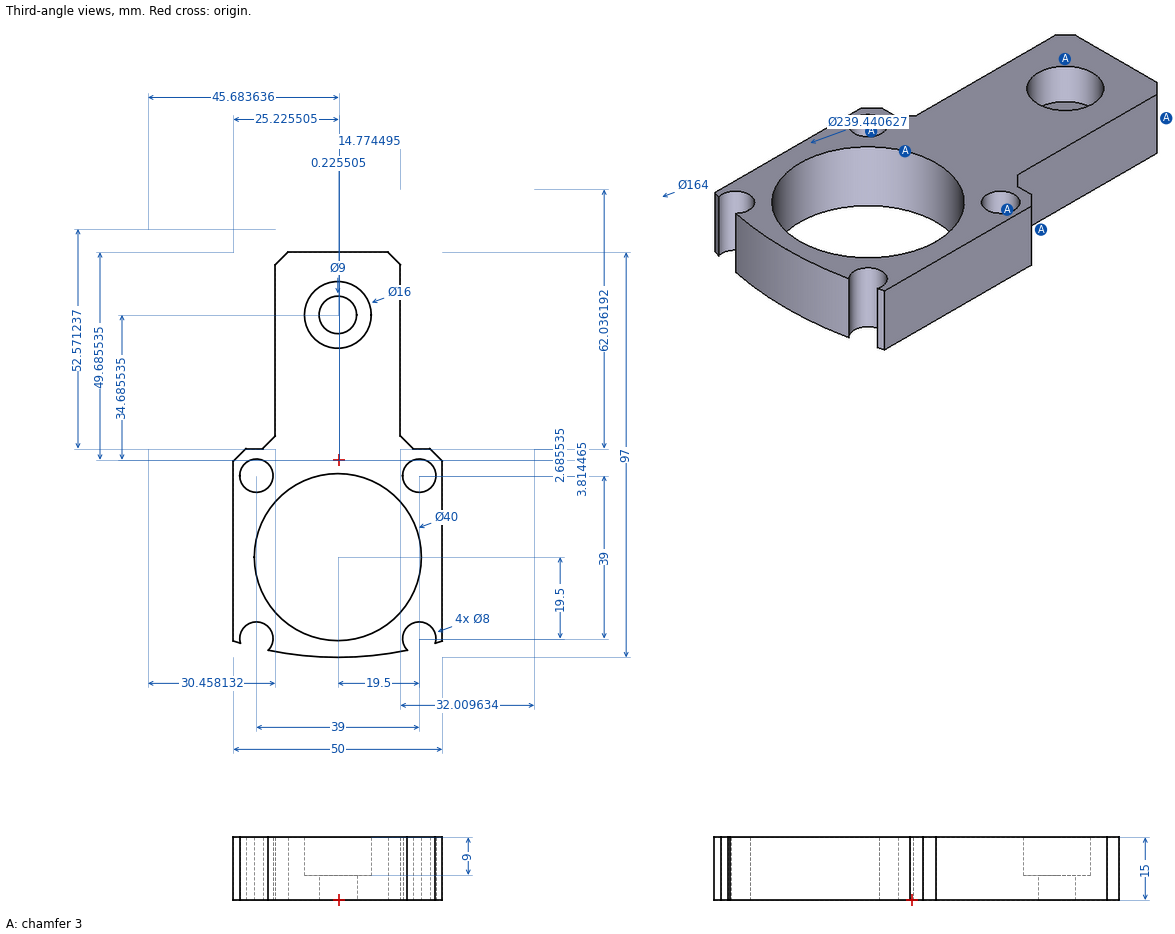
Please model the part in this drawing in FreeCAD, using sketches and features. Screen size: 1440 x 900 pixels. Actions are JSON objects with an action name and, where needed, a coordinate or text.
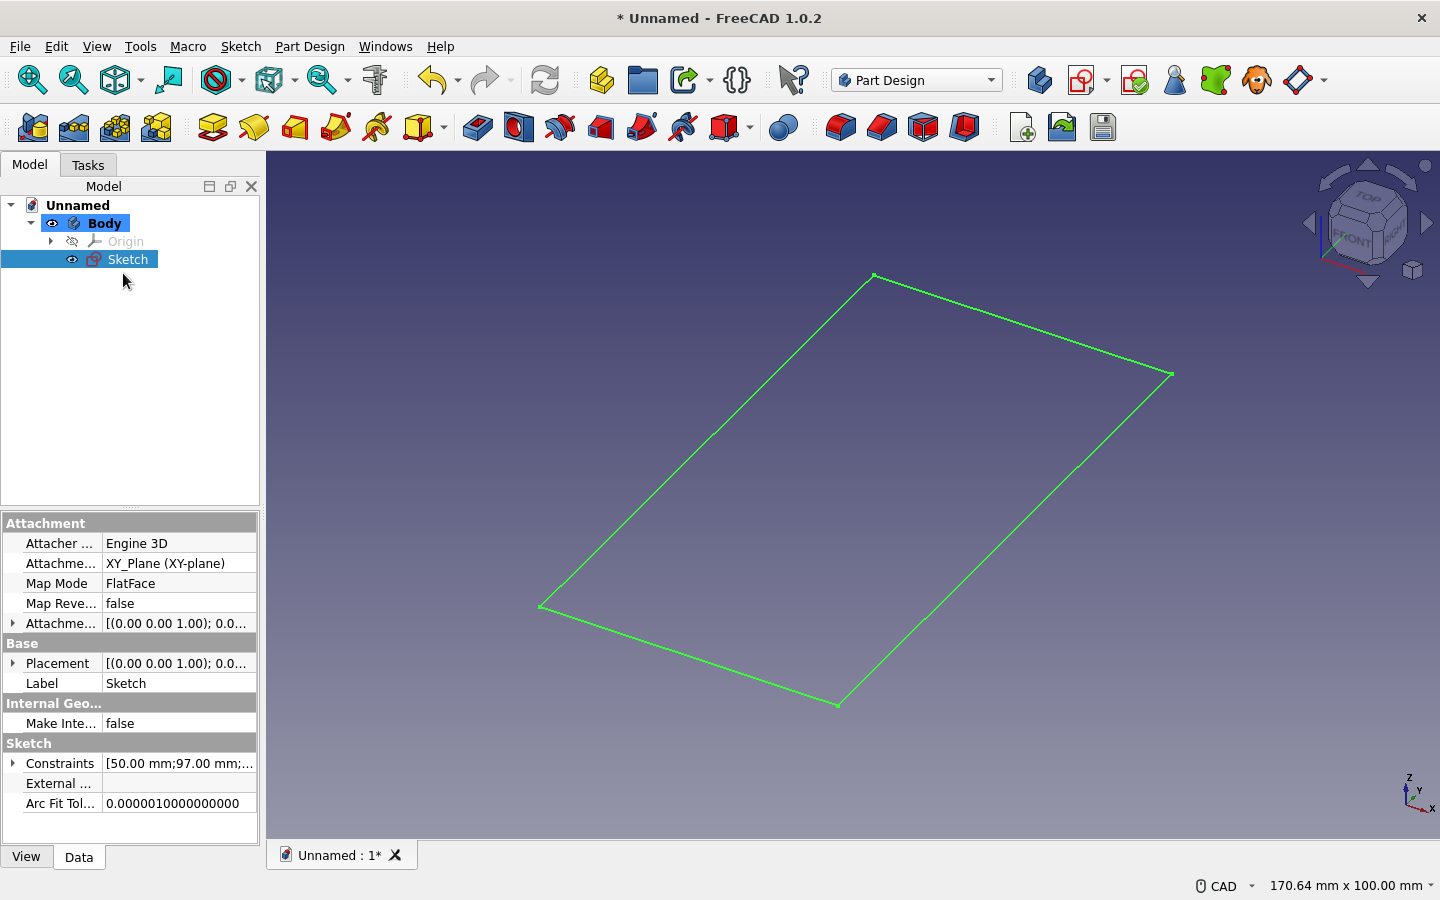
{"action": "left_click", "coordinate": [213, 128]}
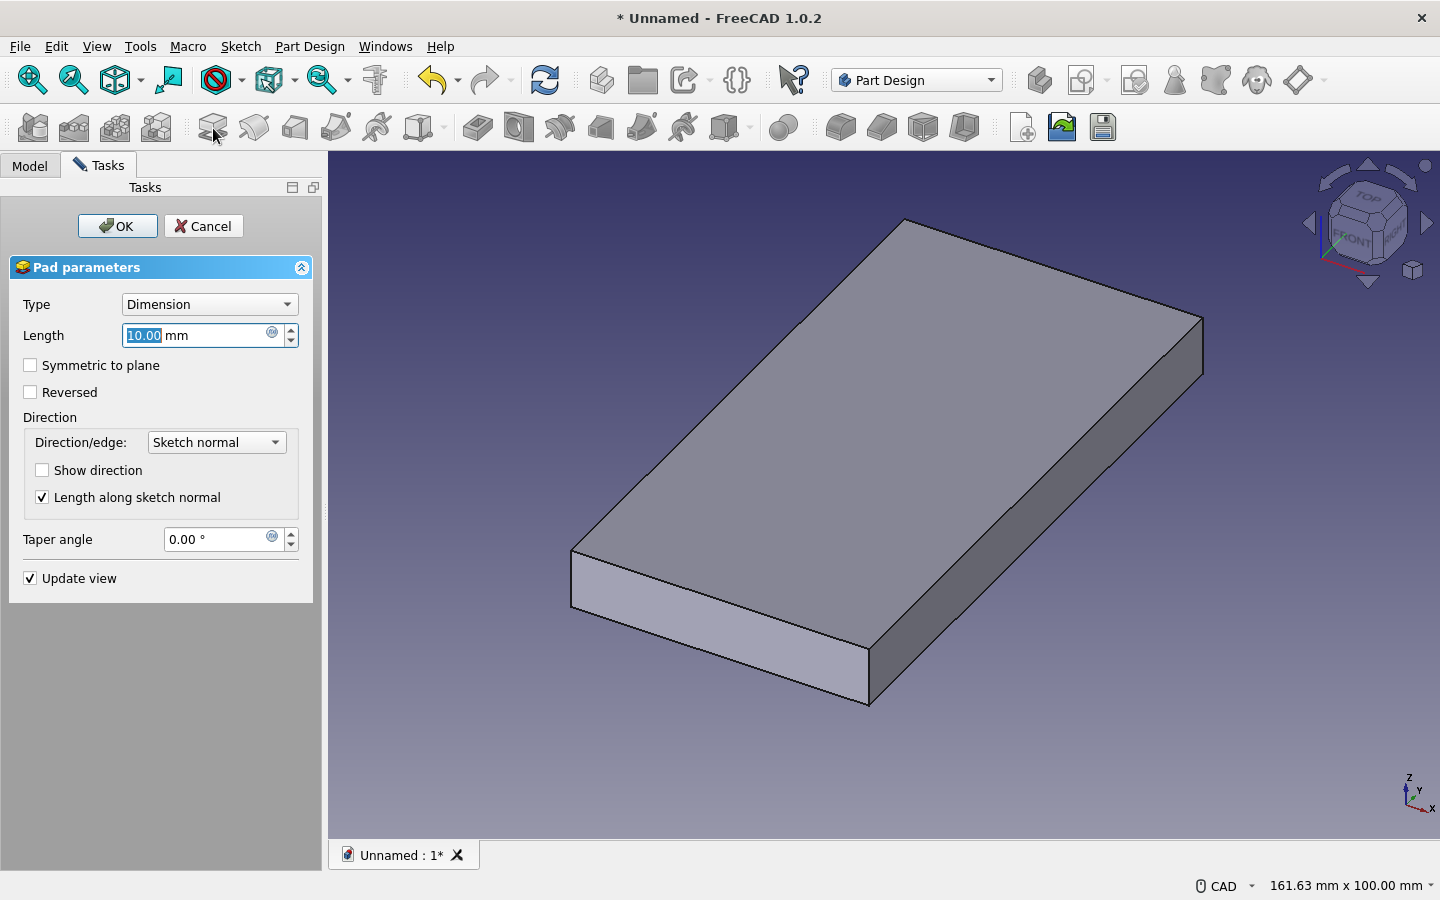
{"action": "type", "text": "15"}
{"action": "key", "text": "Tab"}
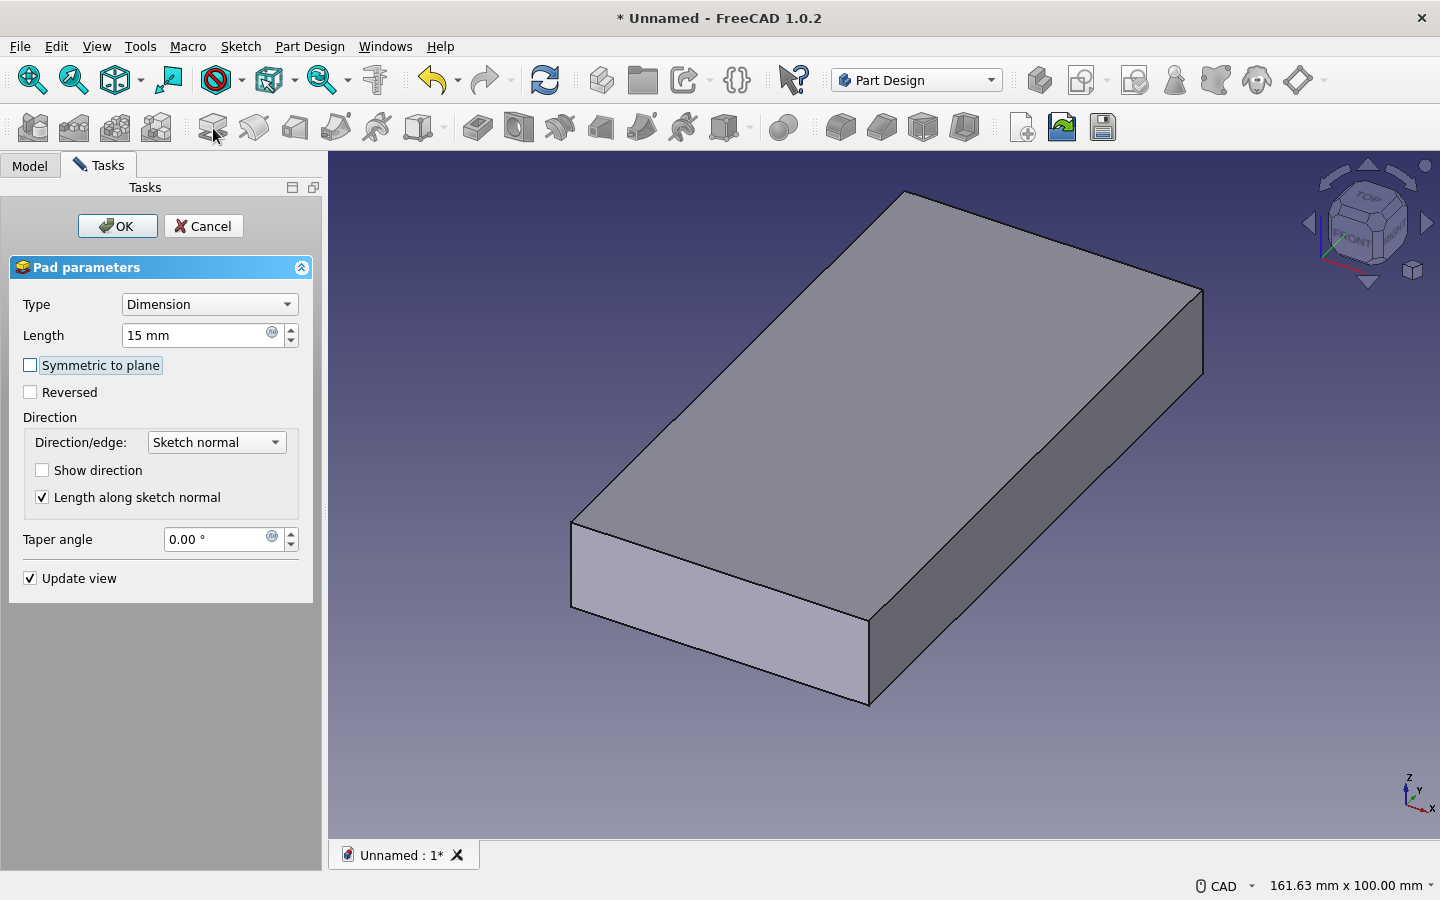
{"action": "left_click", "coordinate": [118, 226]}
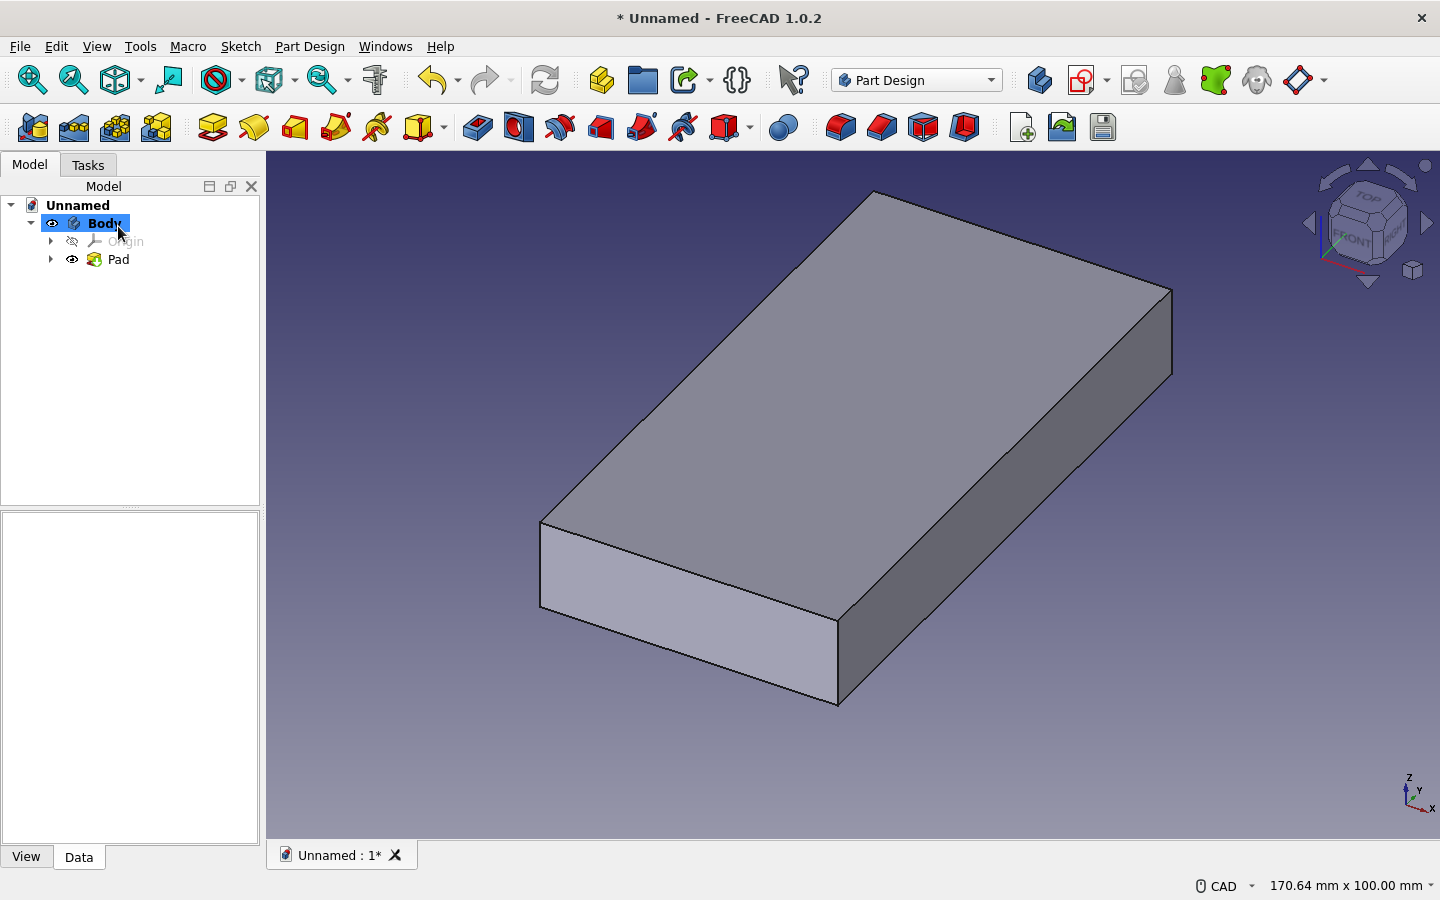
{"action": "left_click", "coordinate": [903, 358]}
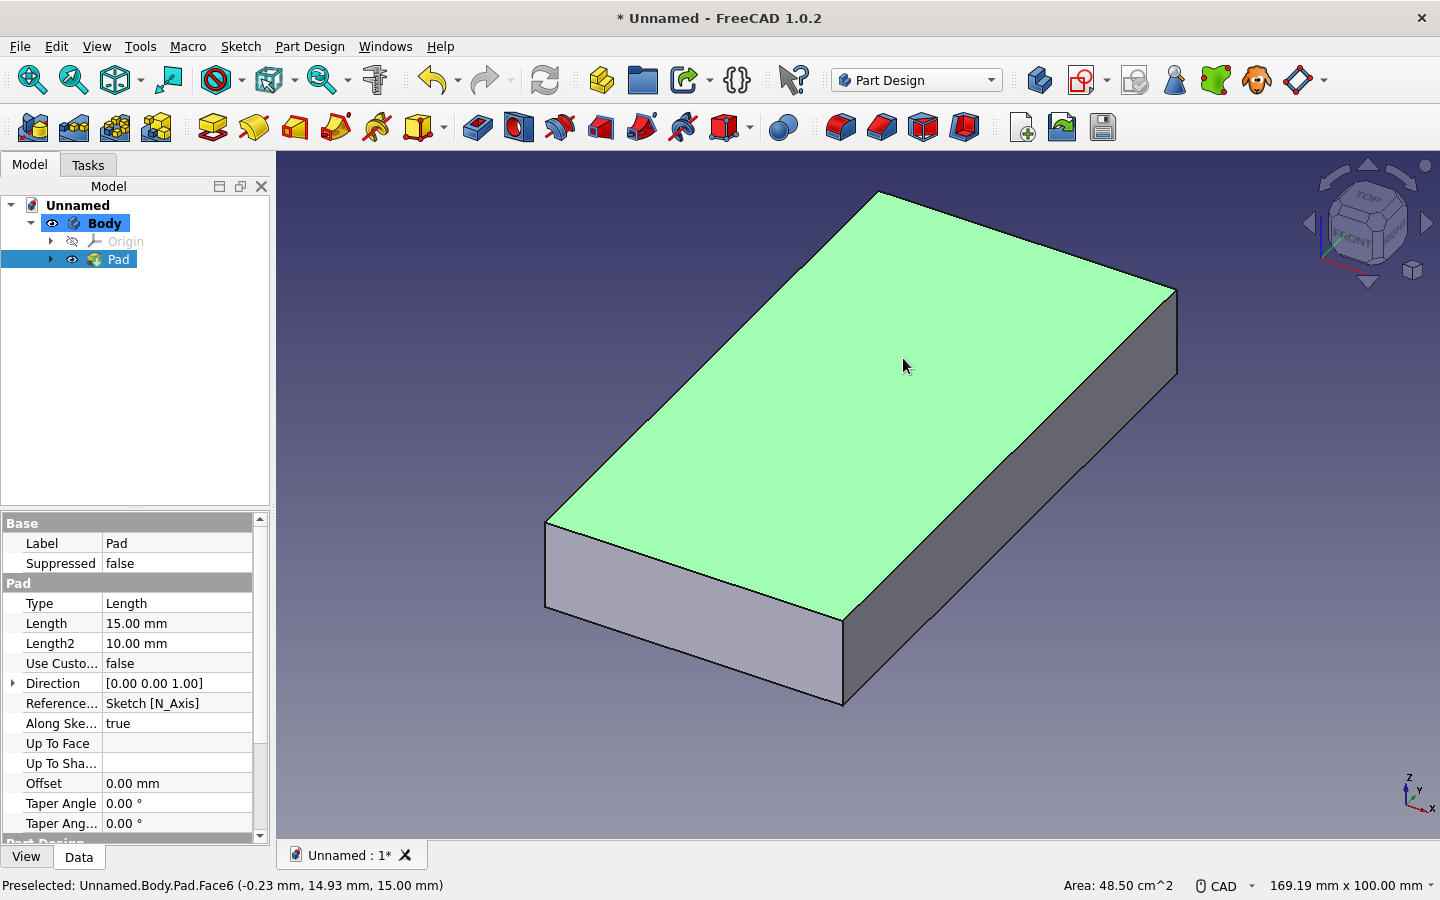
{"action": "left_click", "coordinate": [1080, 80]}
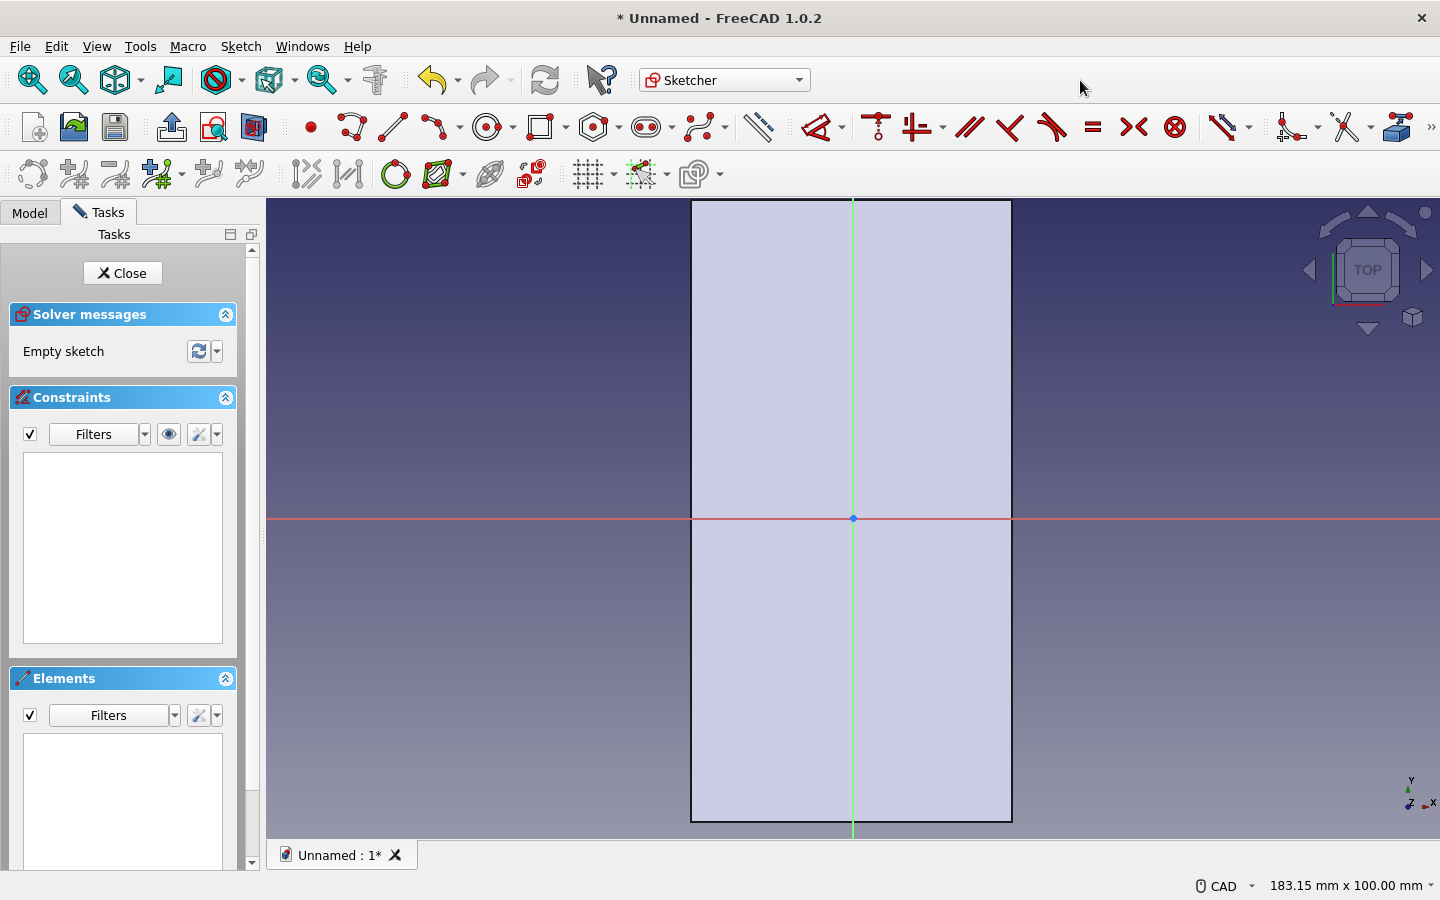
{"action": "scroll", "coordinate": [874, 226], "scroll_direction": "up", "scroll_amount": 7}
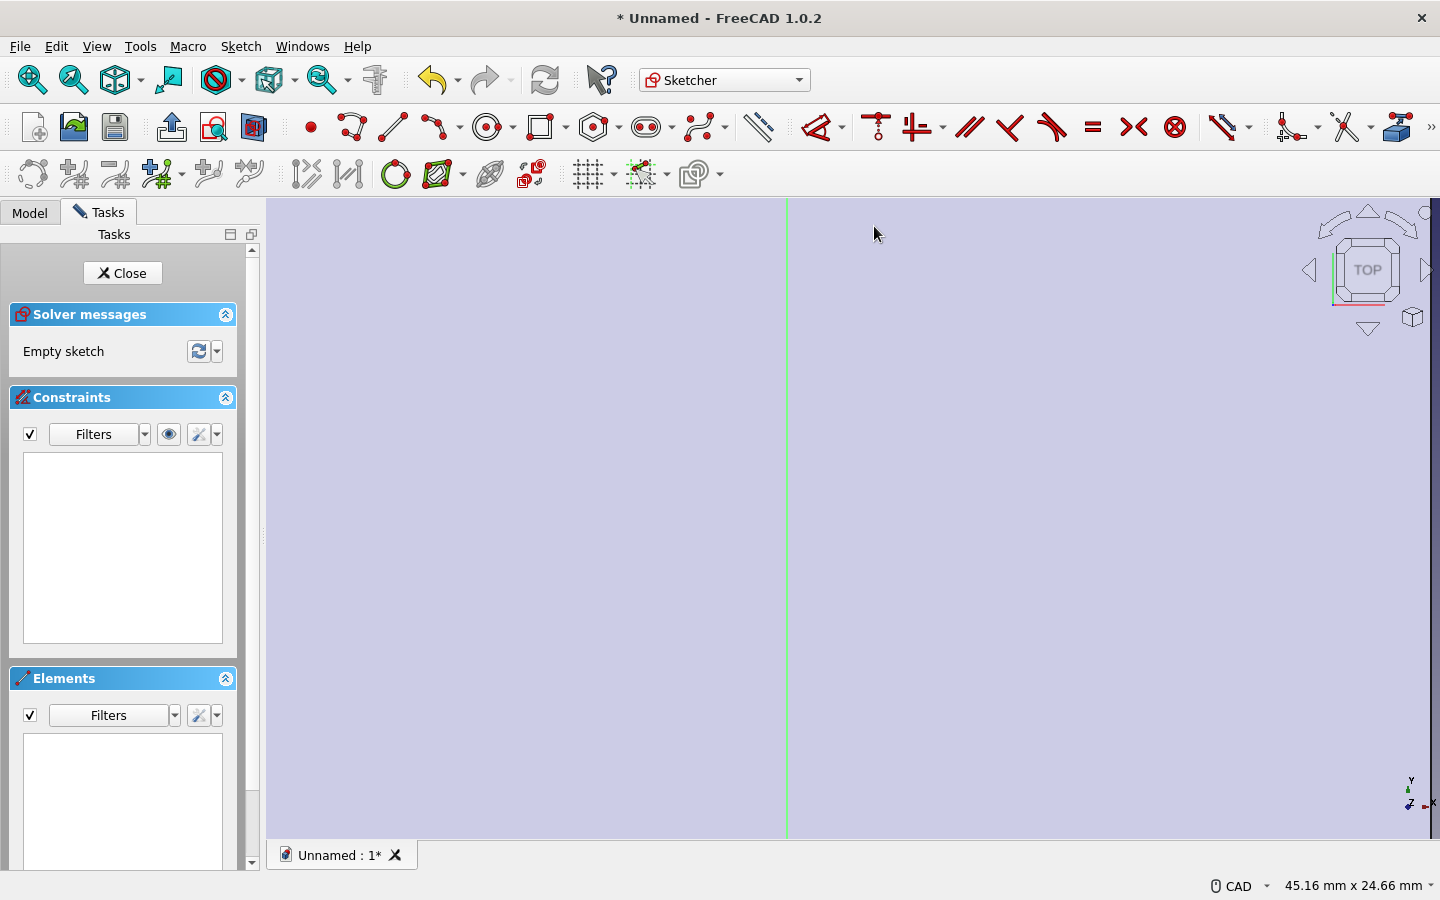
{"action": "key", "text": "g c"}